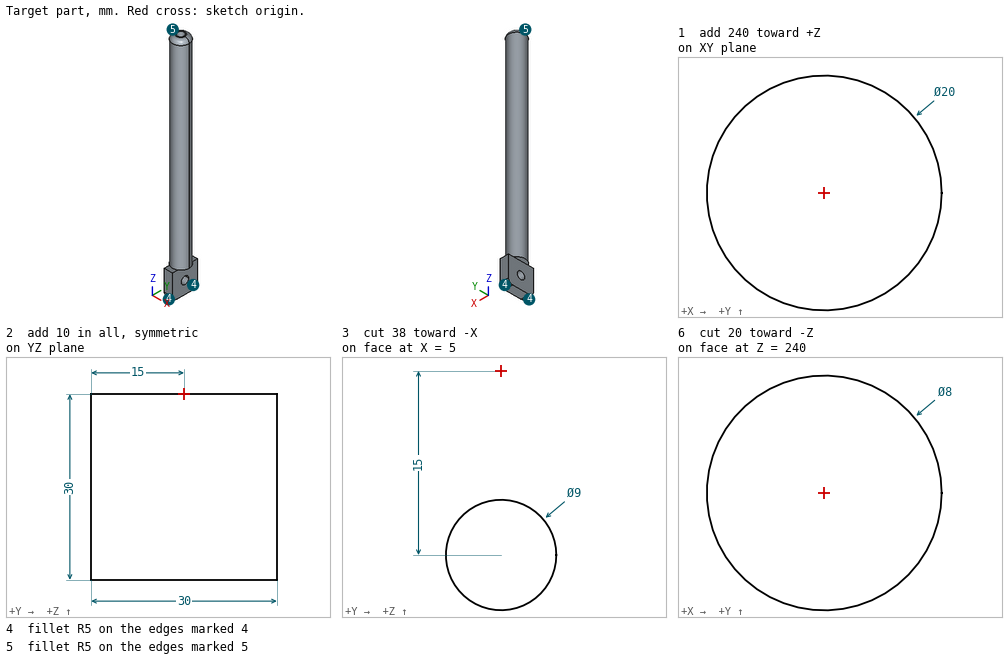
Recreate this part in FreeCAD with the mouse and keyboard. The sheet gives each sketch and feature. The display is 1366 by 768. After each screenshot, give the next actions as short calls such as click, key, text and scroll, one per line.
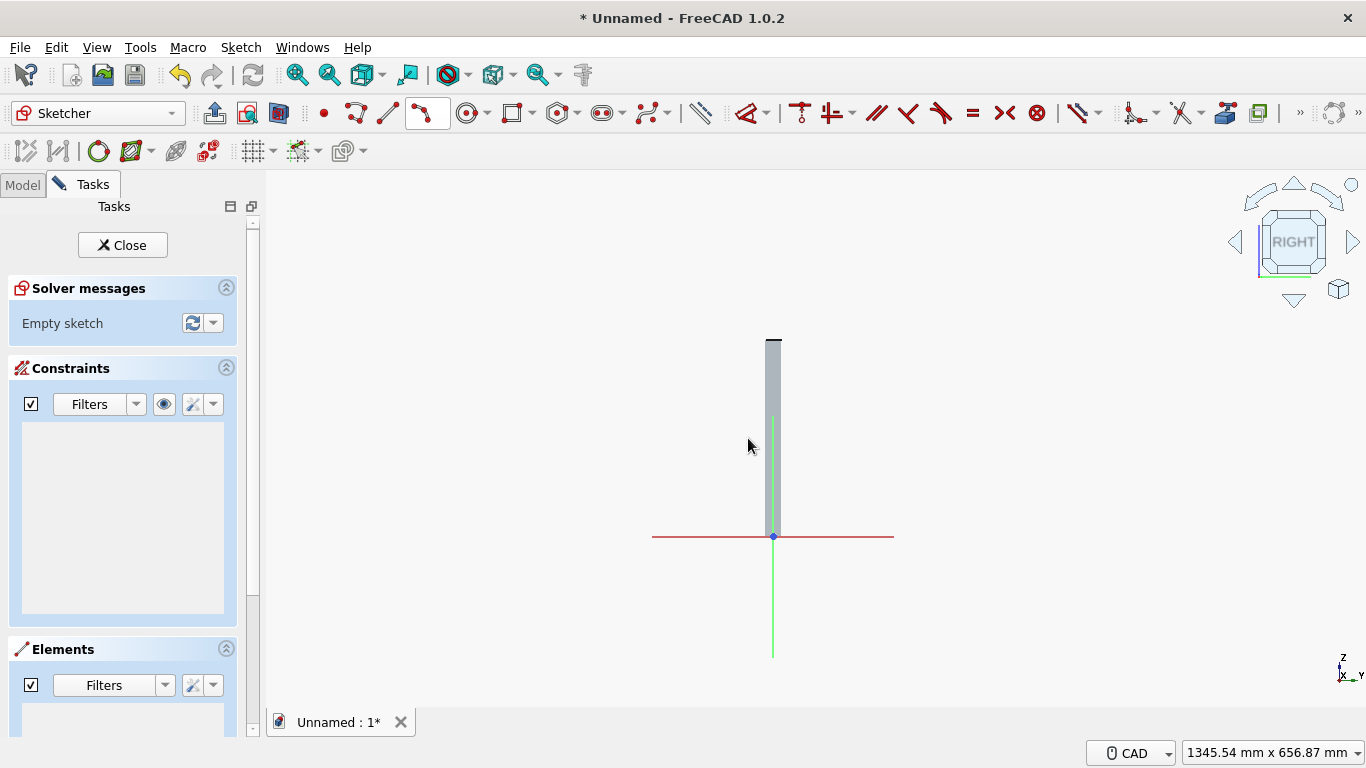
scroll(775, 558, up, 13)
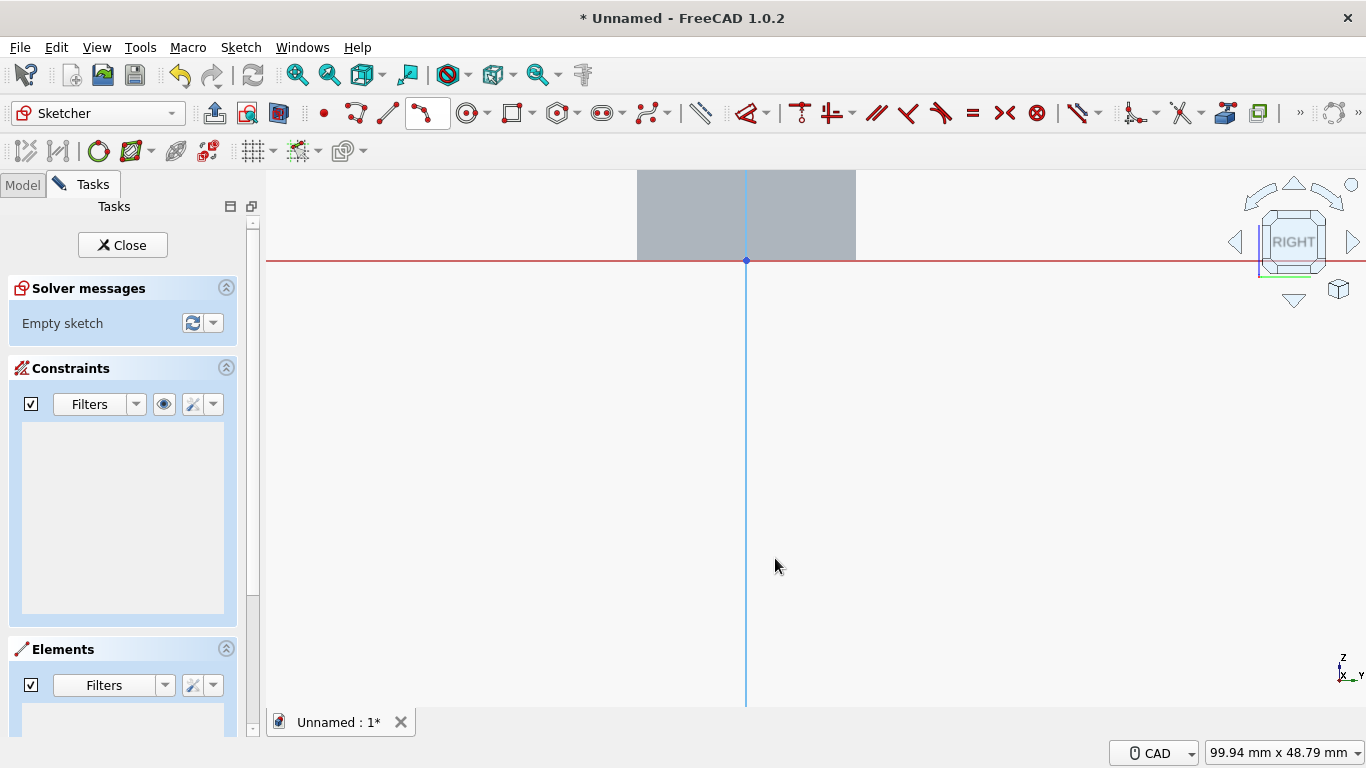
key(g)
key(r)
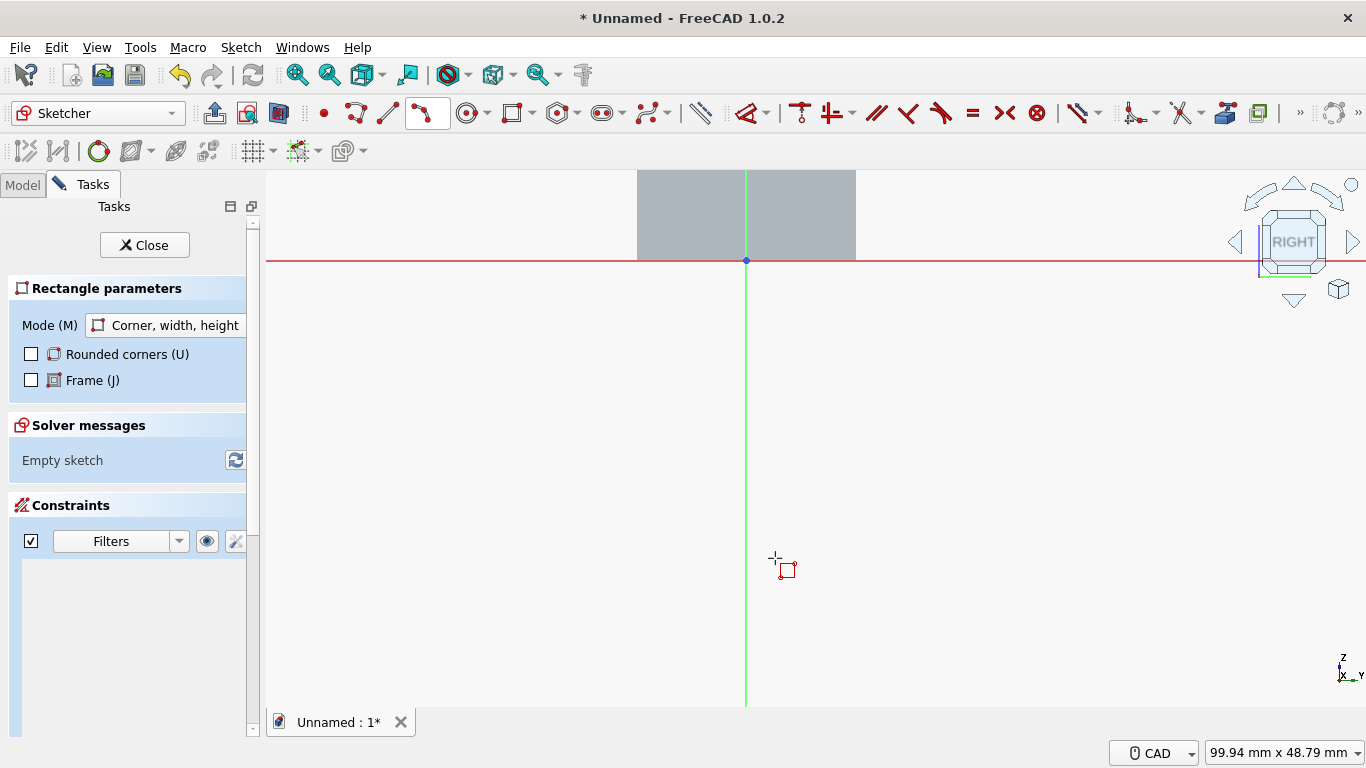
click(581, 261)
click(911, 591)
key(Escape)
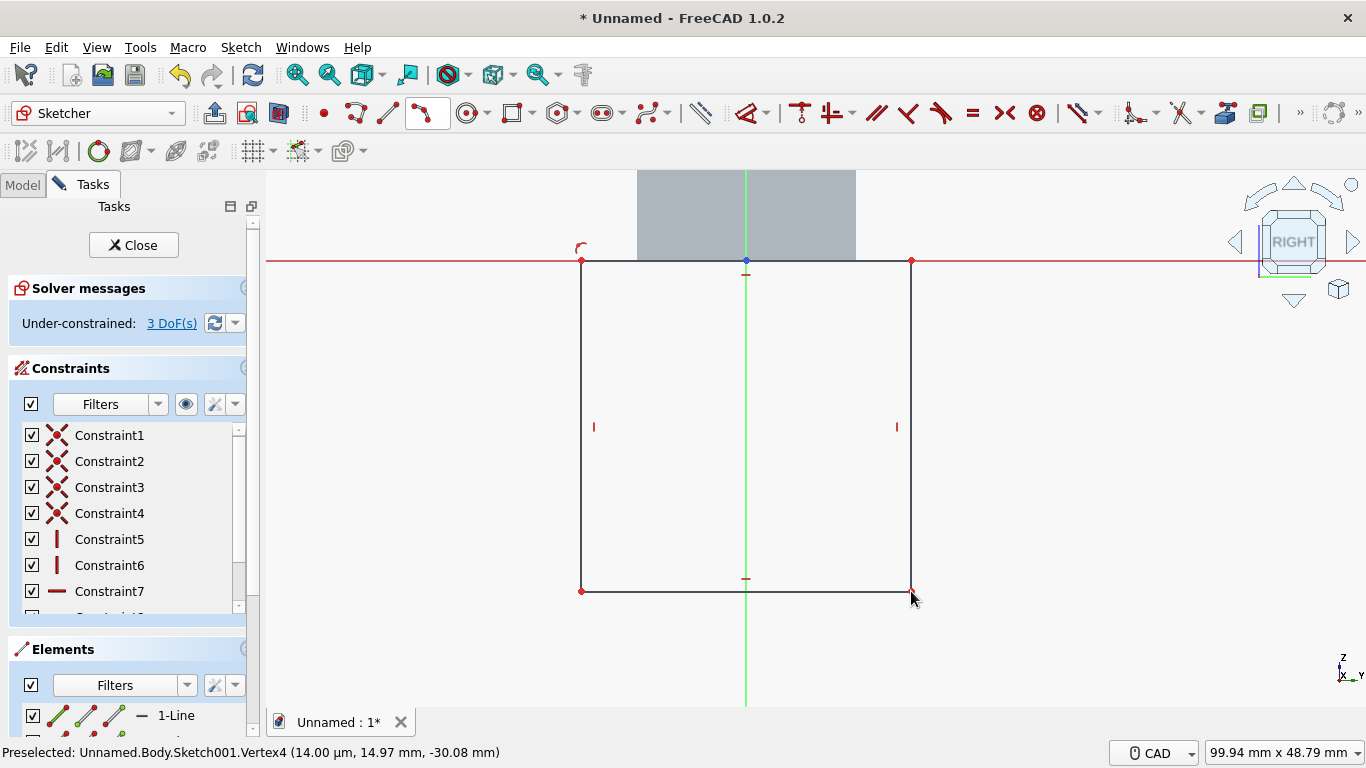
click(746, 114)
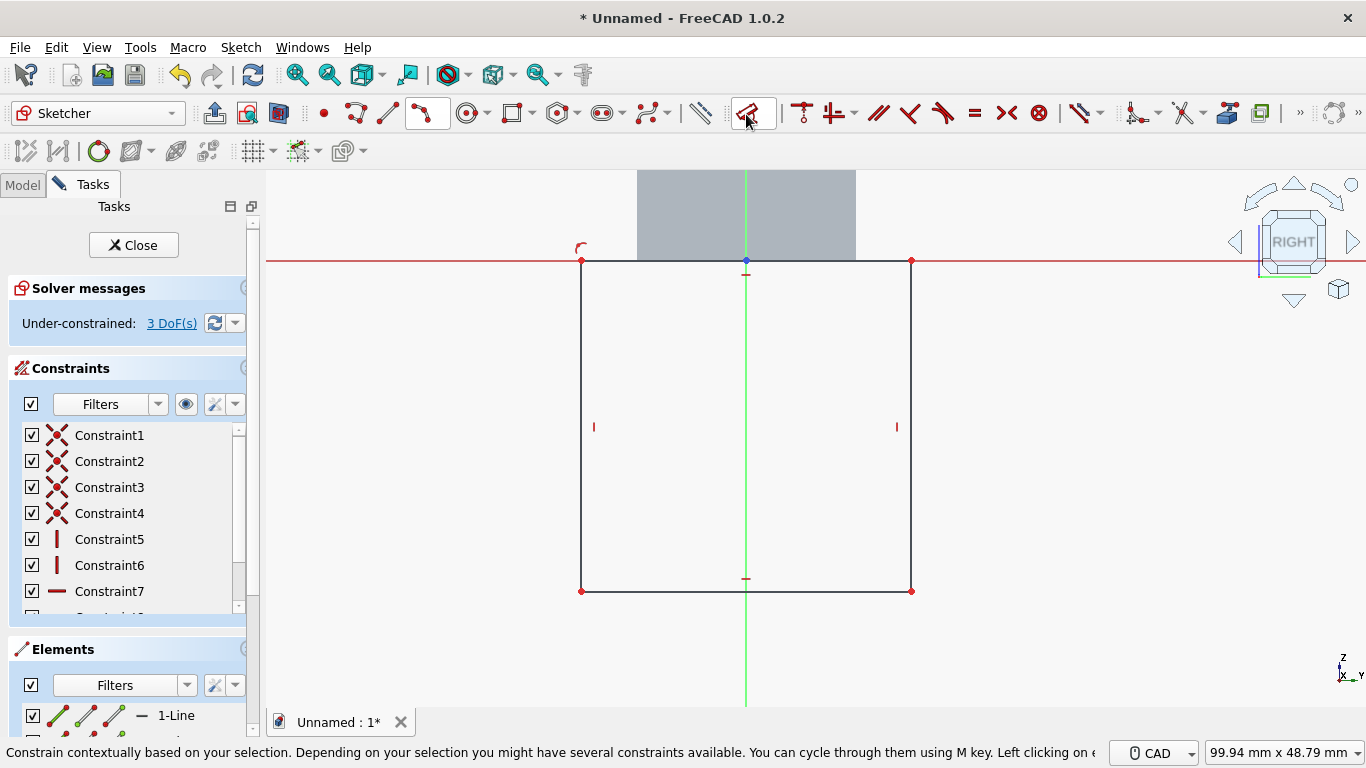
click(581, 360)
click(547, 426)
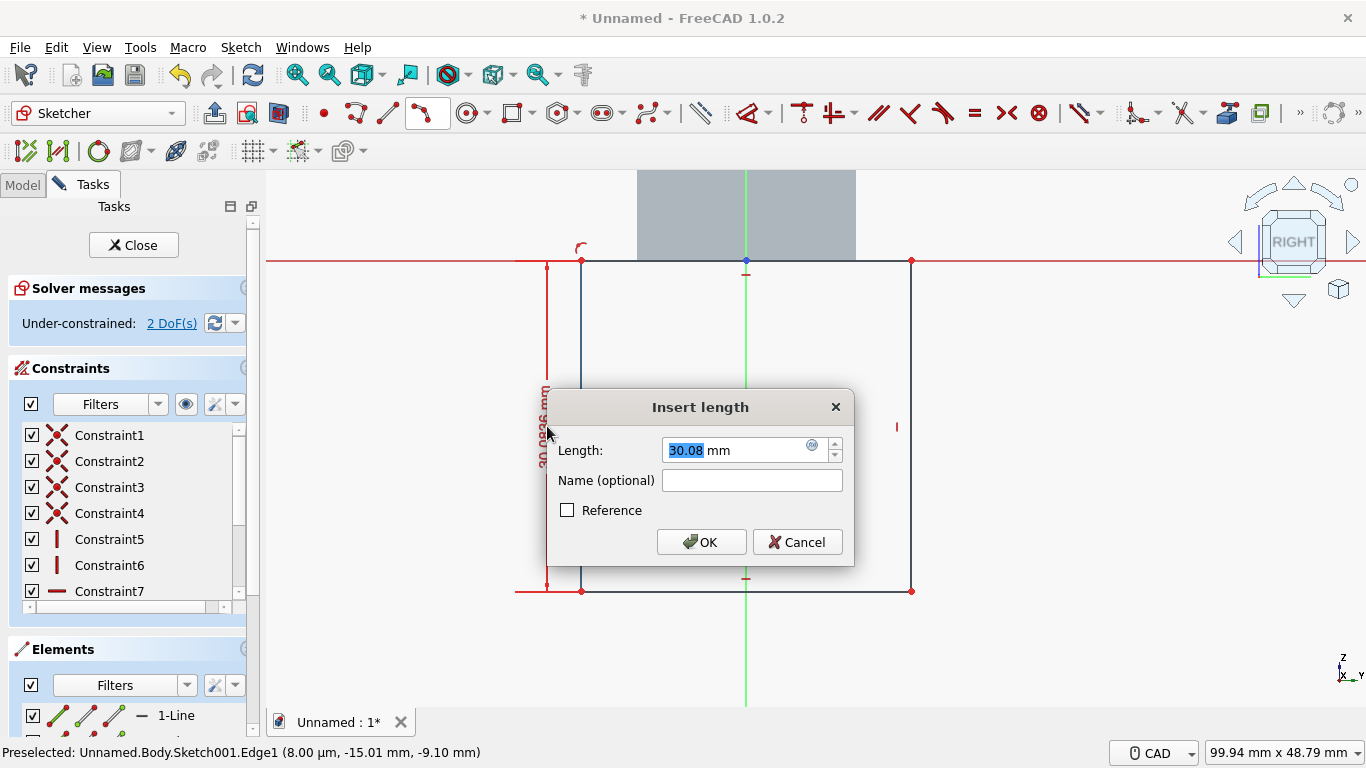
text(30)
key(Return)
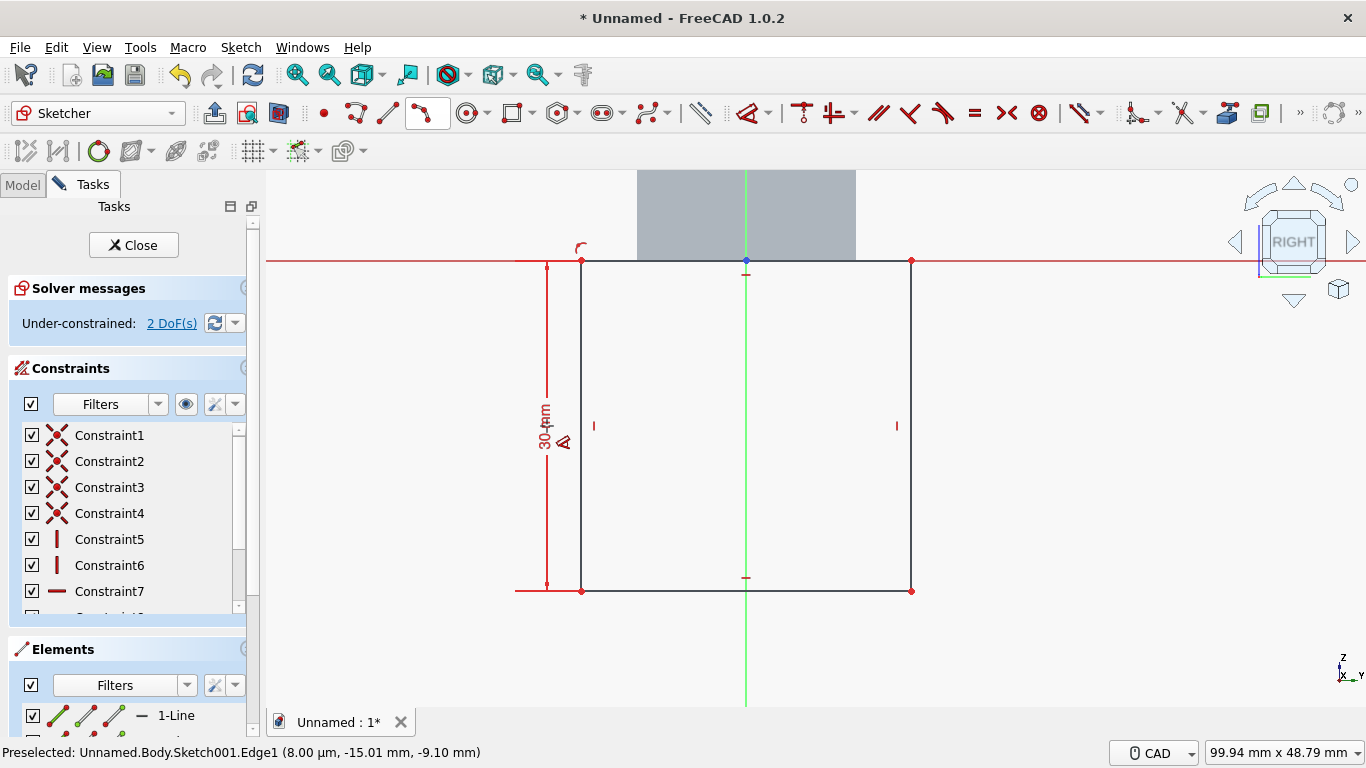
click(680, 591)
click(670, 625)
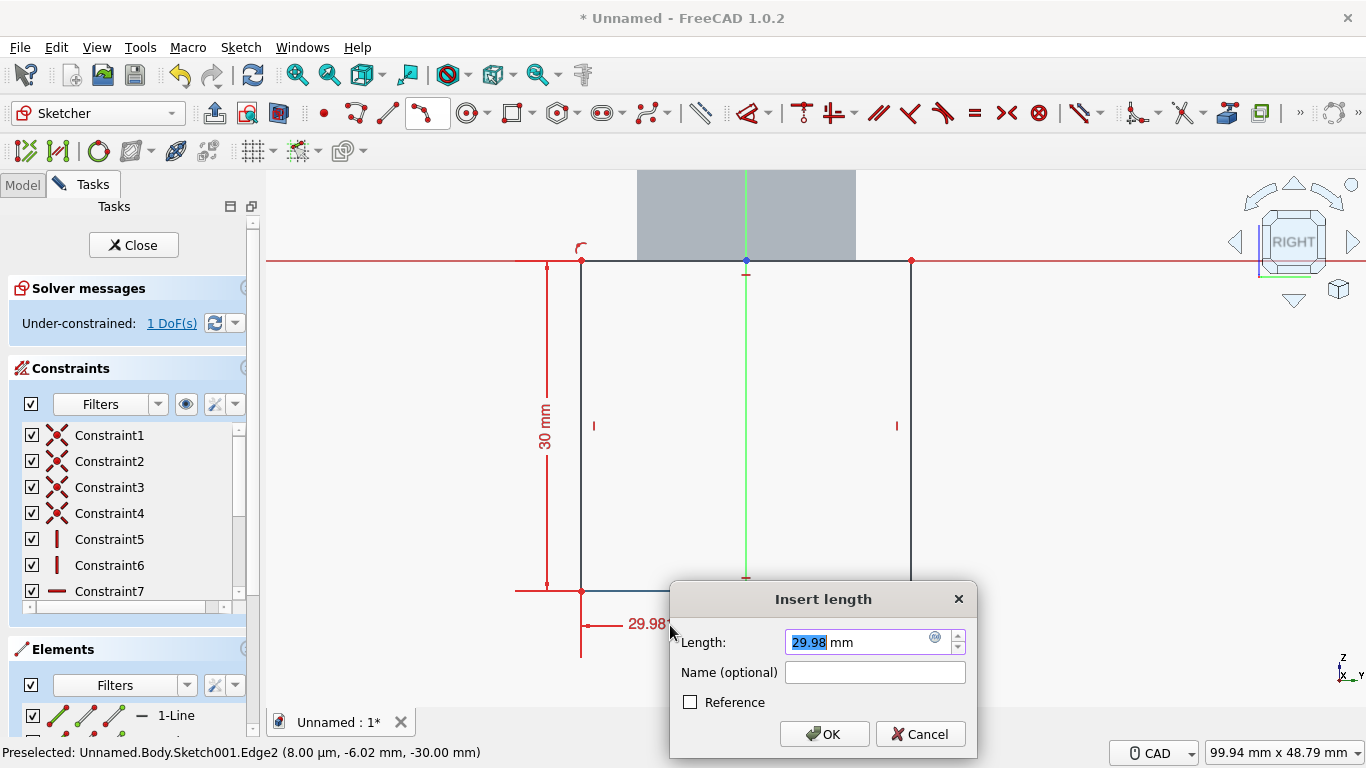
text(30)
key(Return)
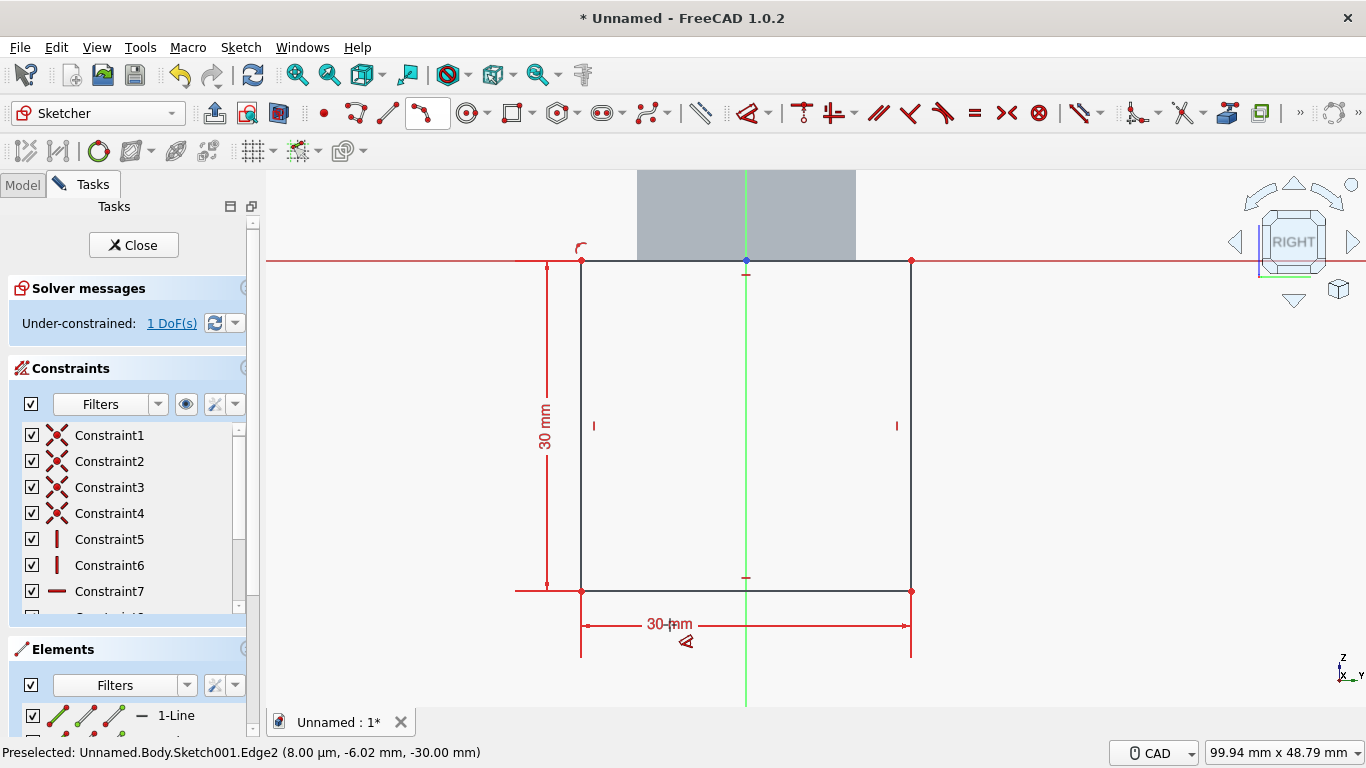
click(581, 261)
click(664, 227)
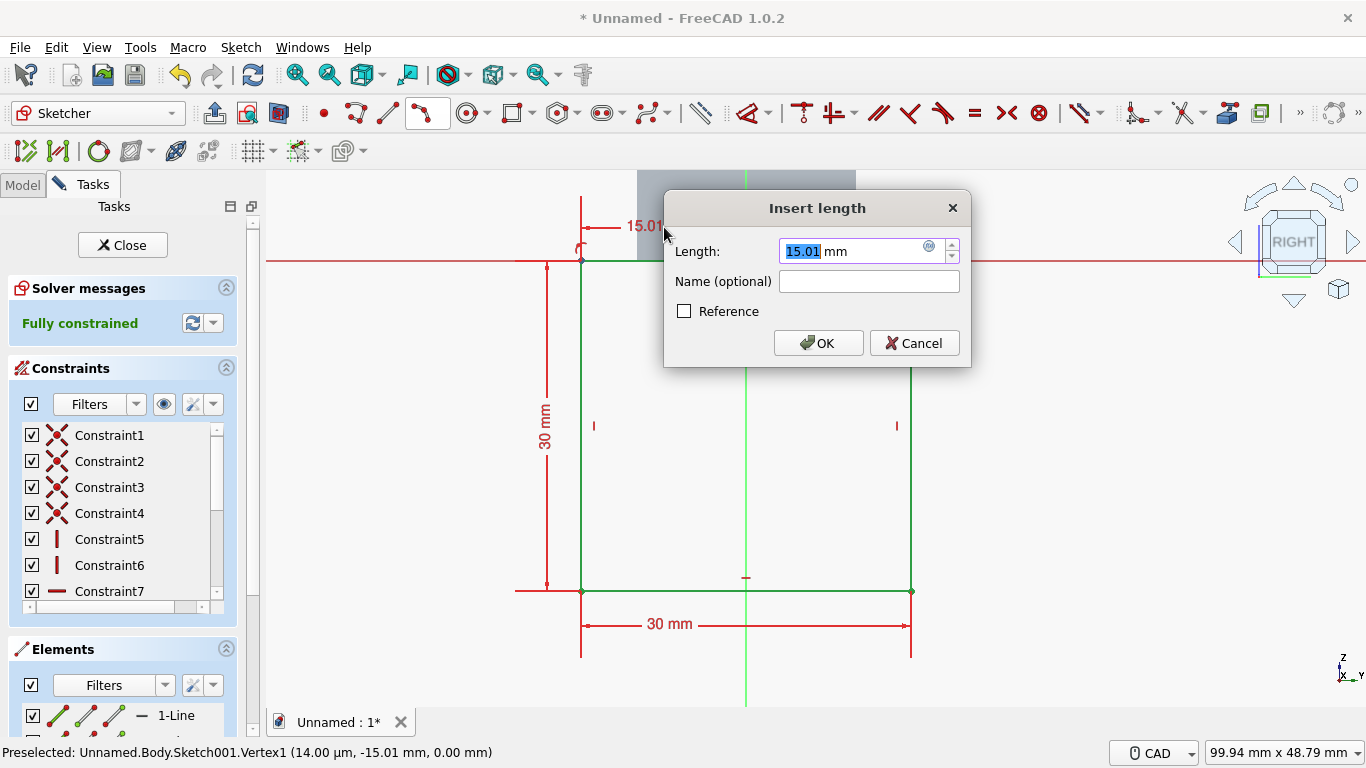
text(15)
key(Return)
key(Escape)